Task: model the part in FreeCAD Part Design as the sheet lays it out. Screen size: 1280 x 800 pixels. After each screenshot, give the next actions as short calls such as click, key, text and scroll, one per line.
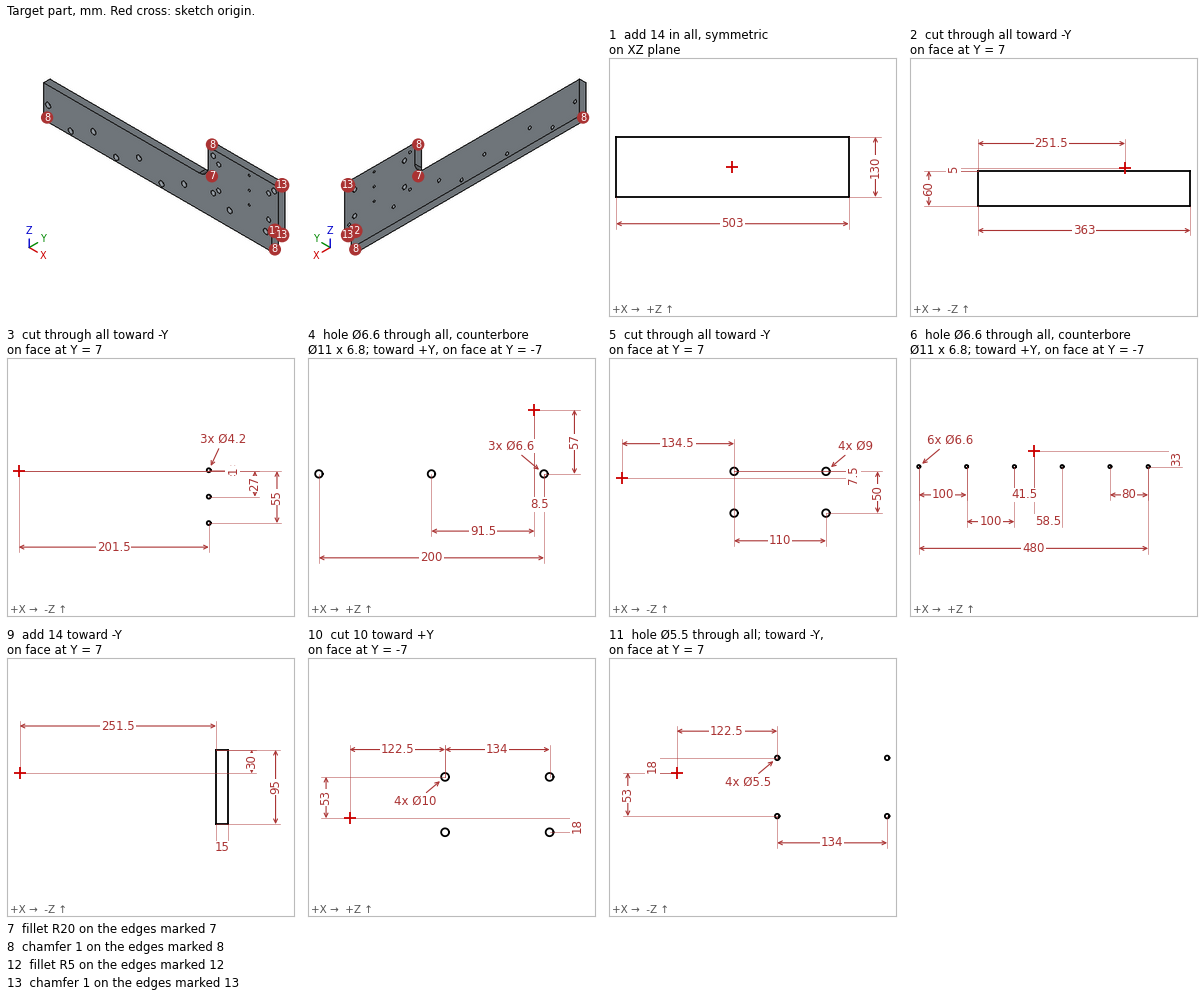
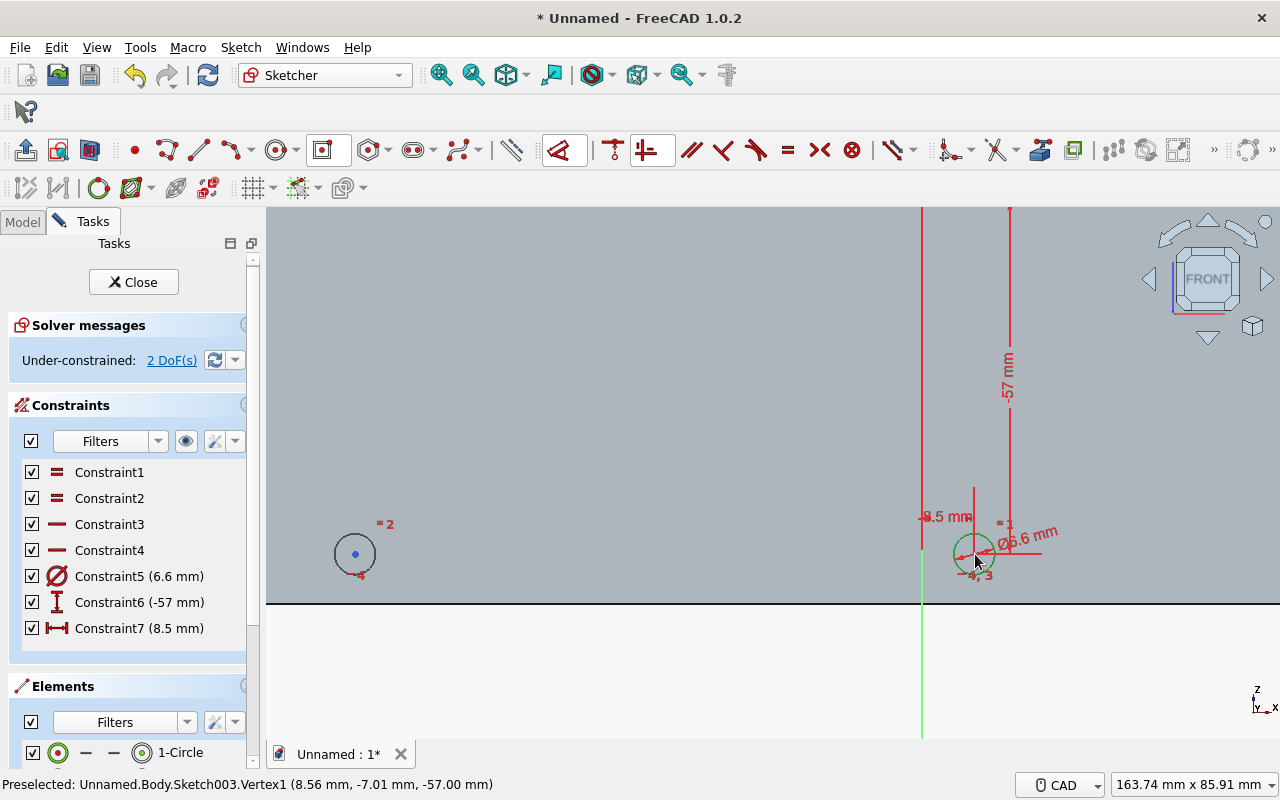
click(355, 554)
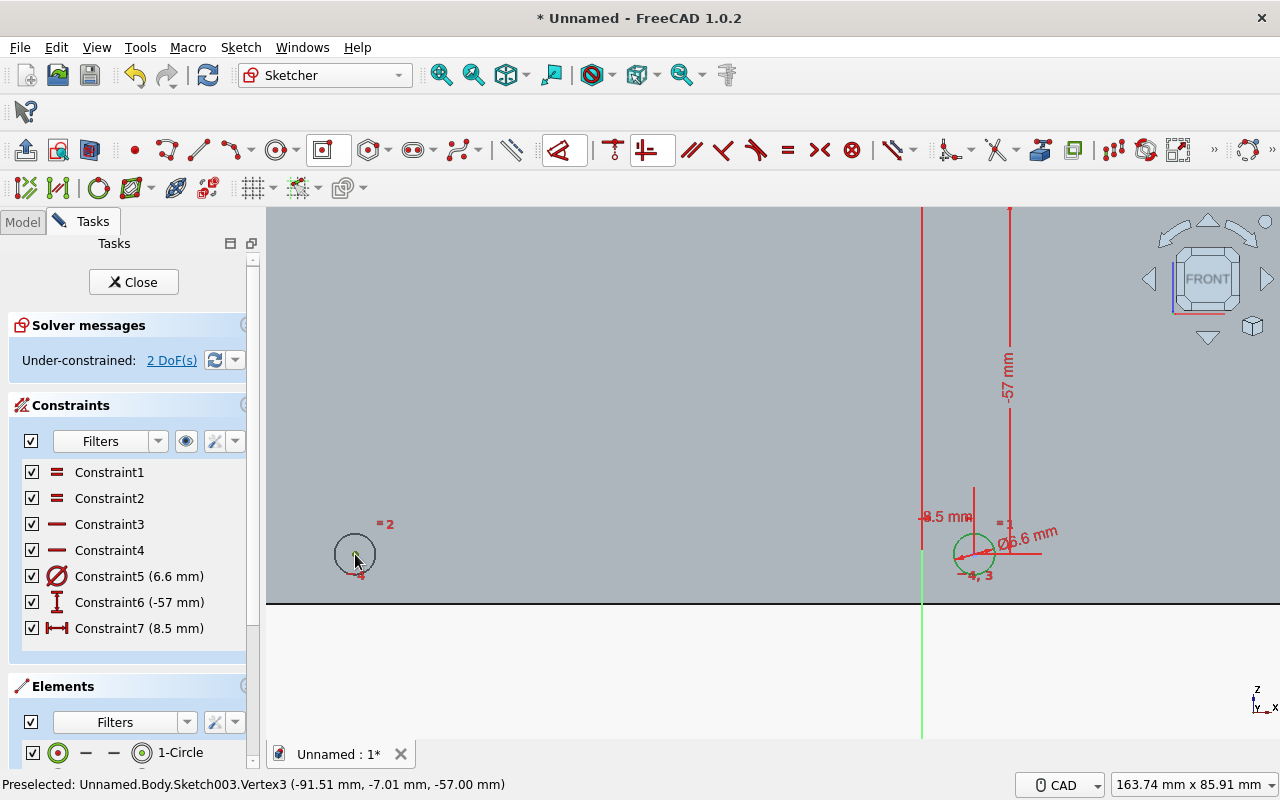
key(l)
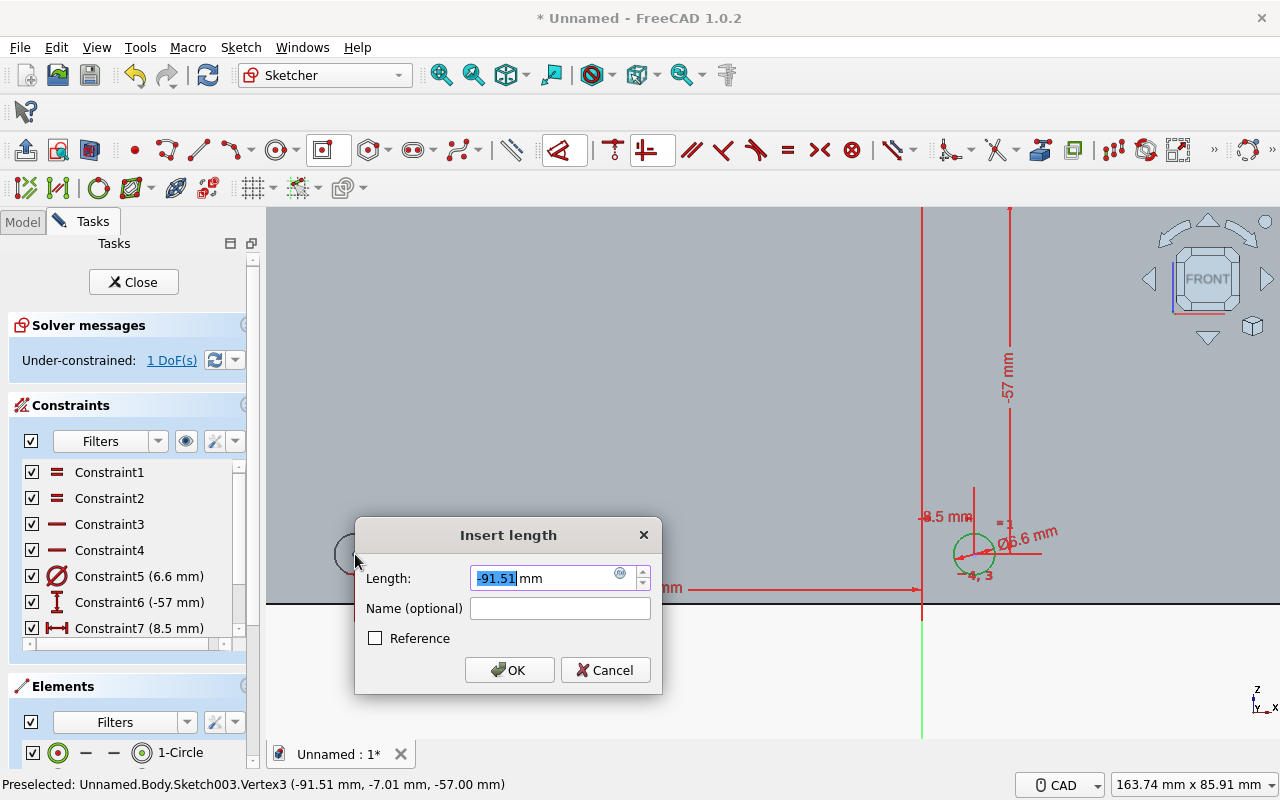
text(-91.5)
key(Return)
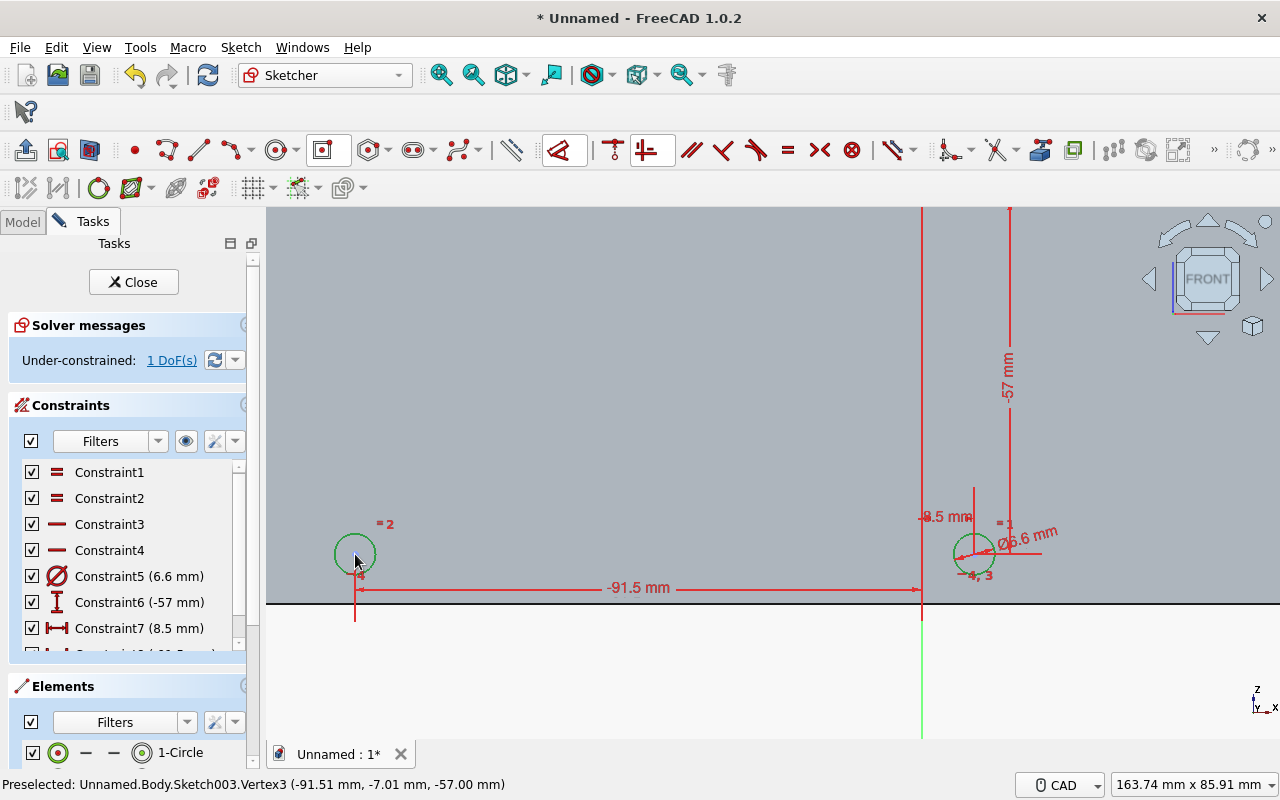
click(974, 554)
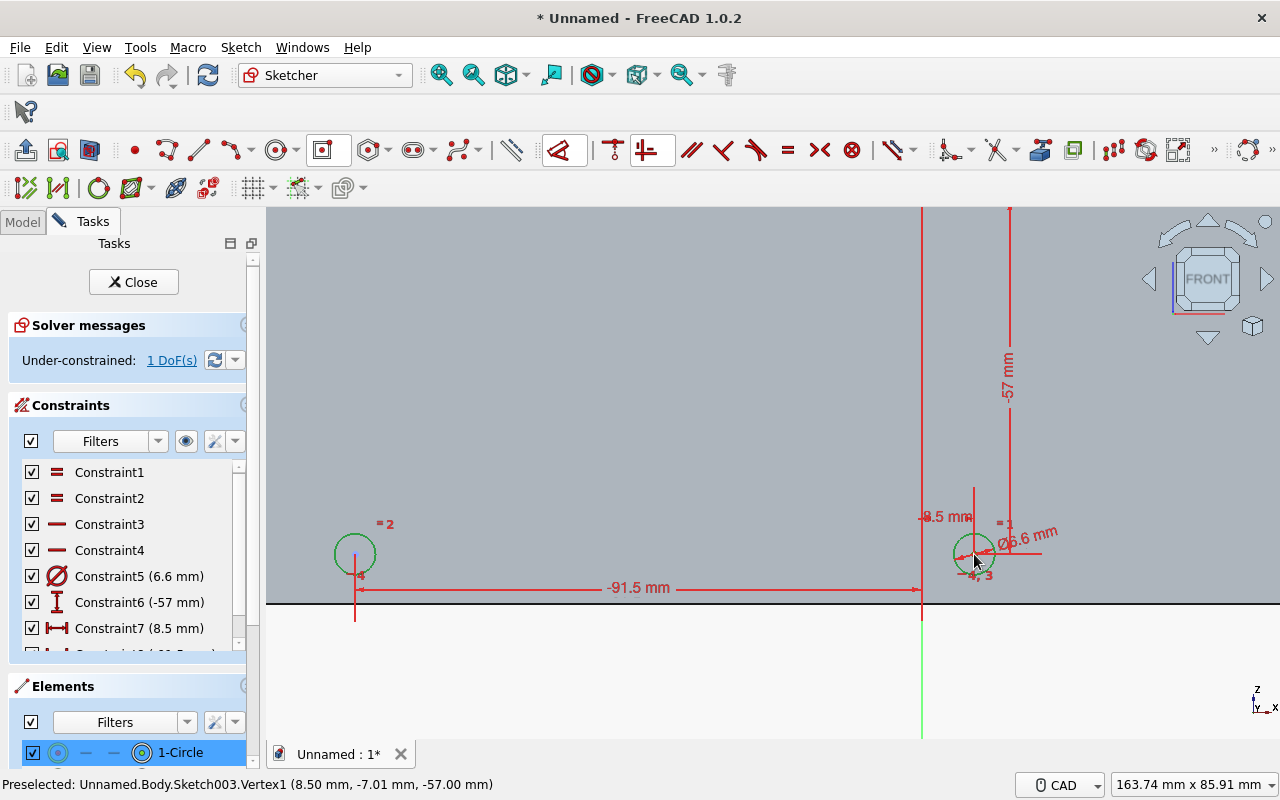
scroll(990, 542, down, 4)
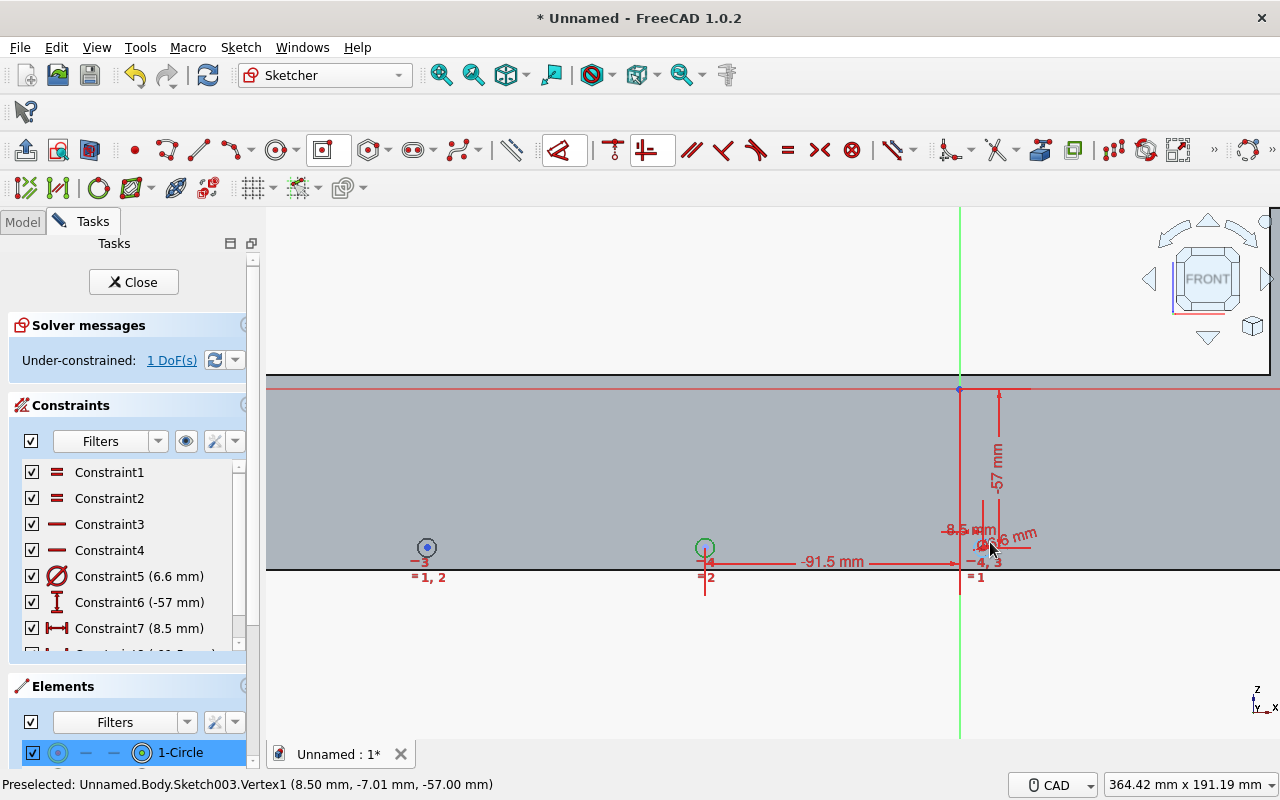
click(427, 548)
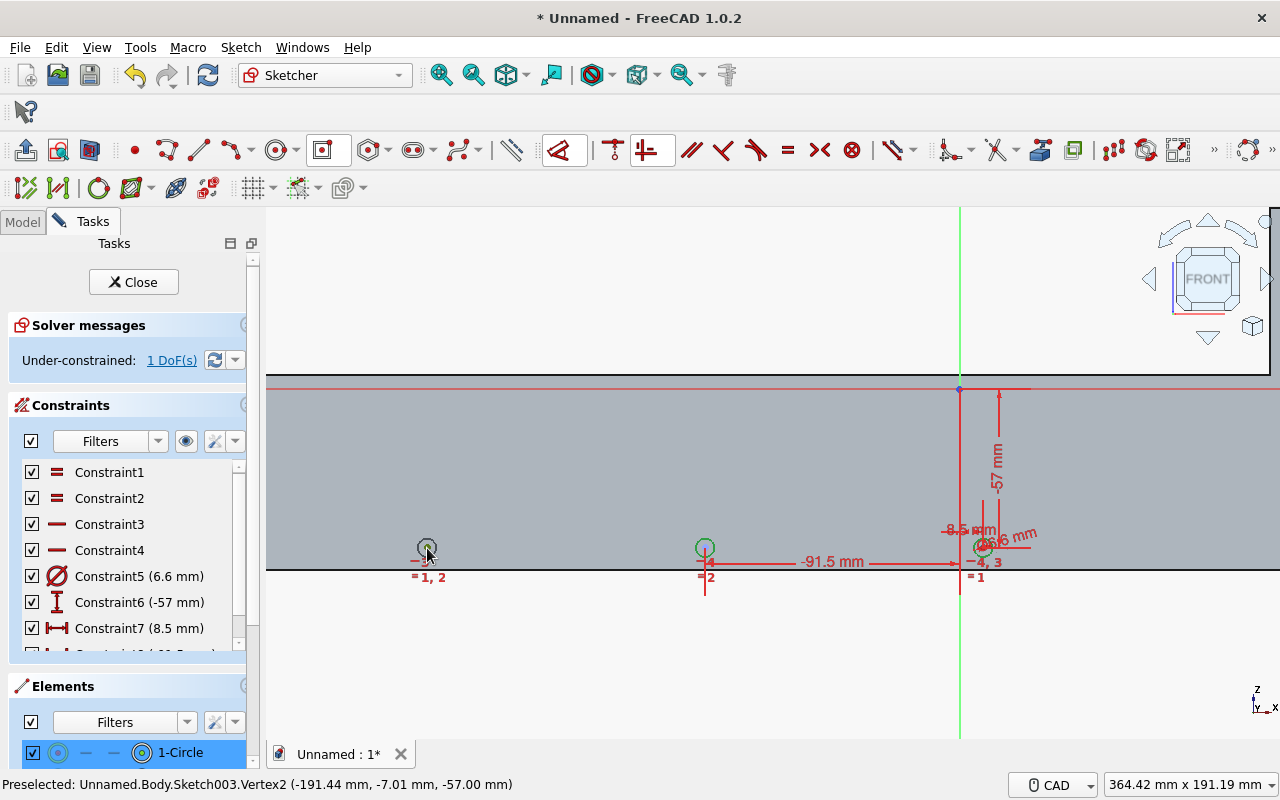
key(l)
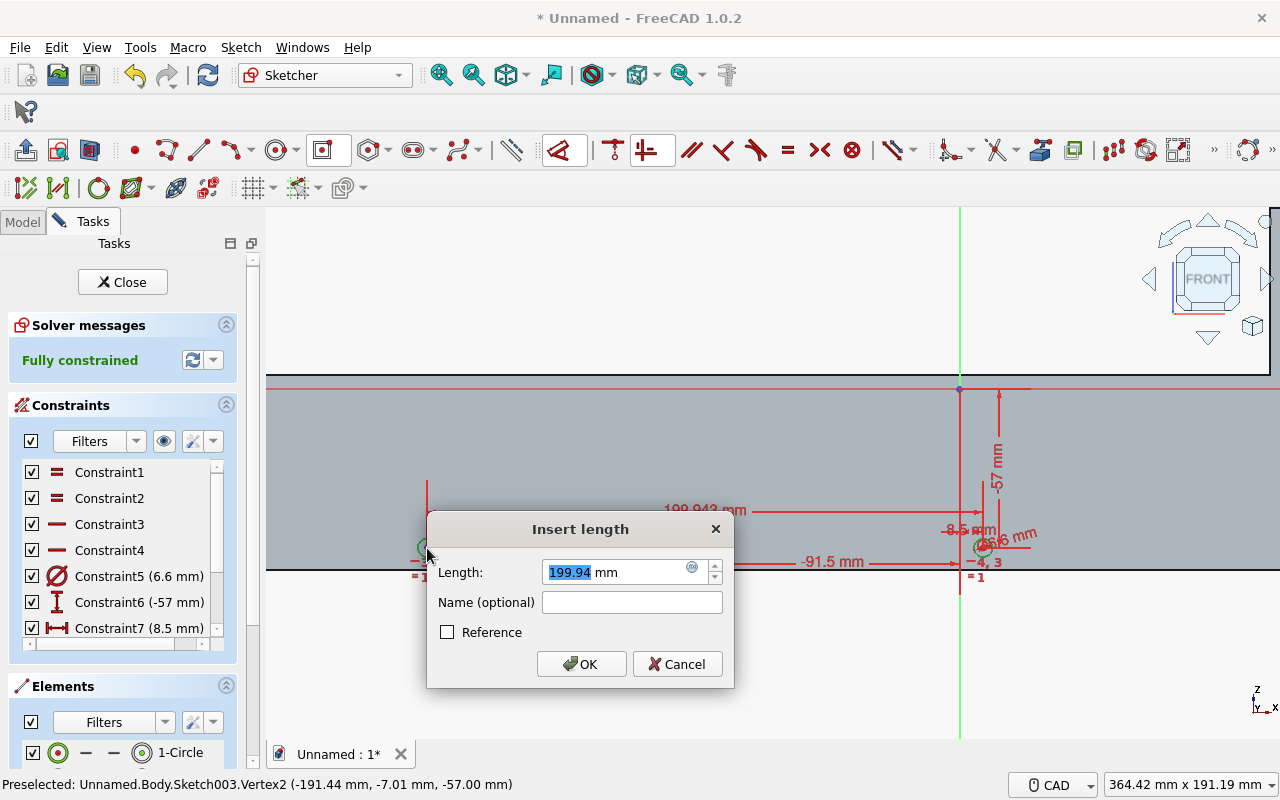
text(200)
key(Return)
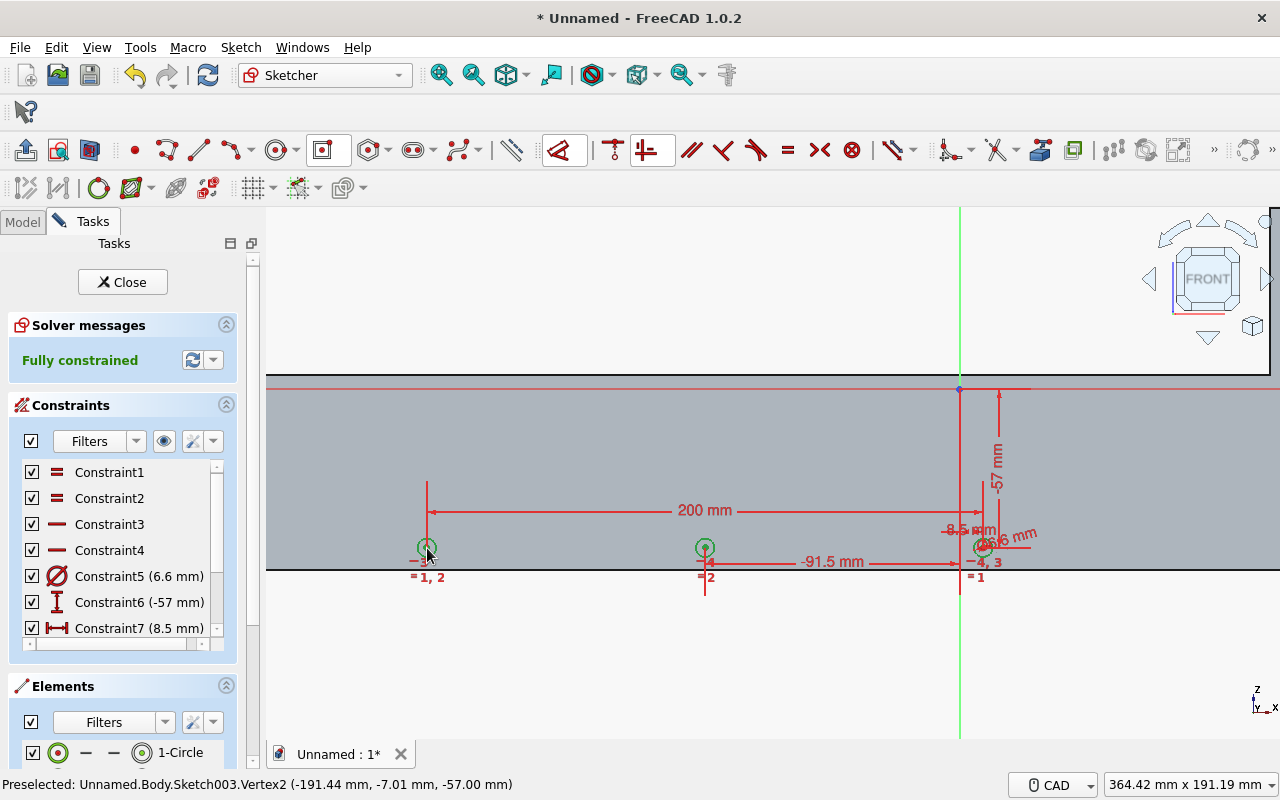
click(123, 282)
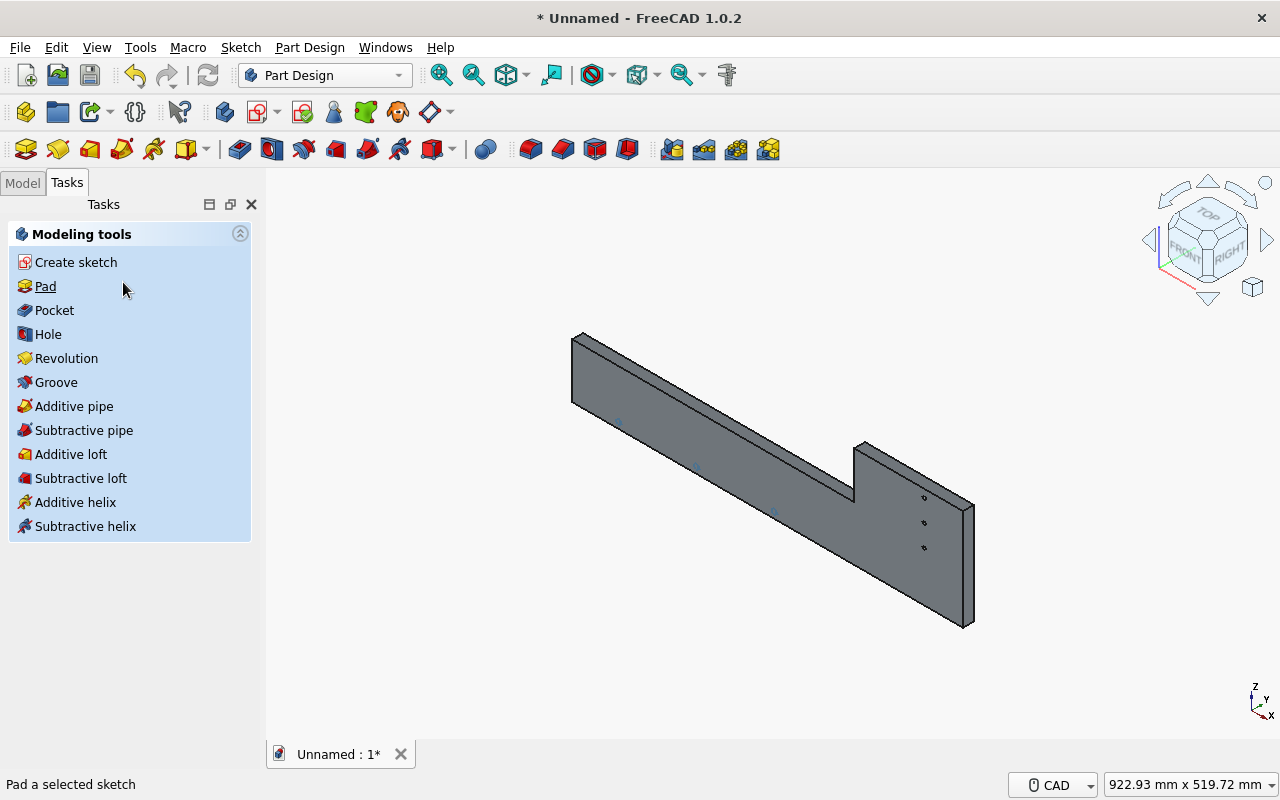
click(272, 150)